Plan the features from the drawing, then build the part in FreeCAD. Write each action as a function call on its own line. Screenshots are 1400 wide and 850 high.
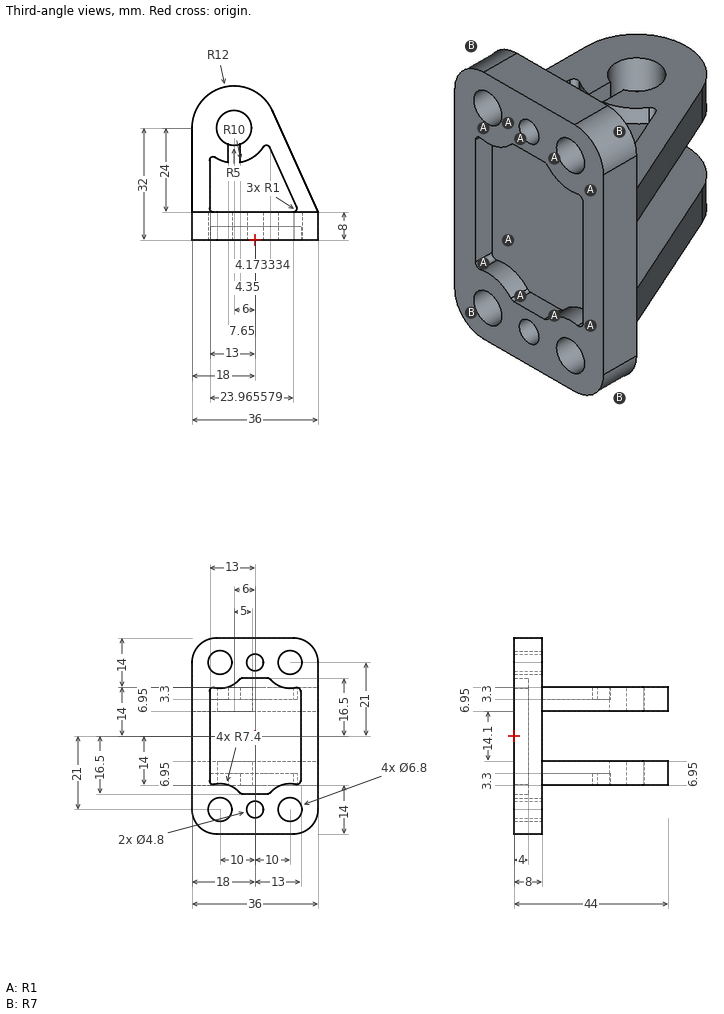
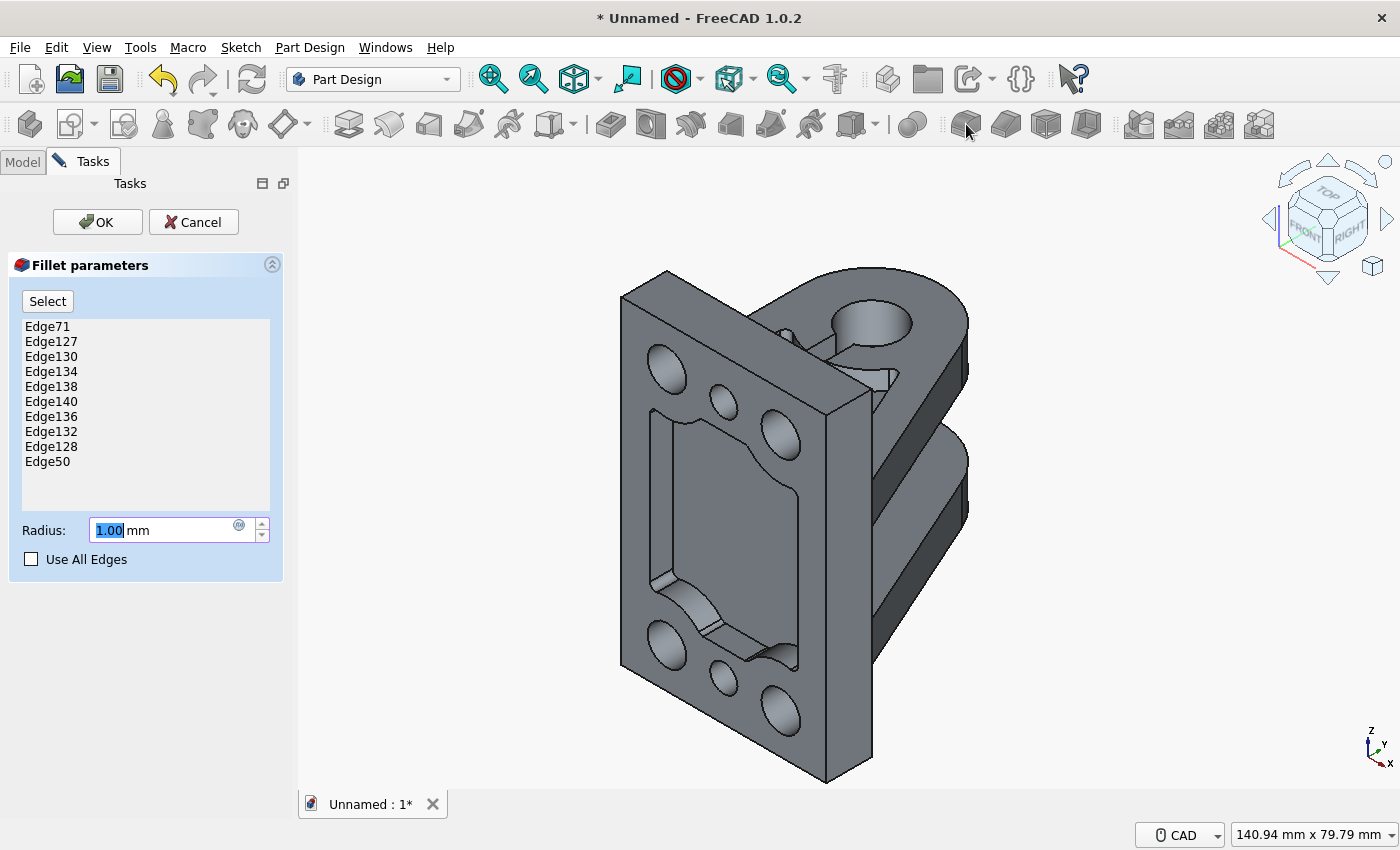
text(1)
key(Tab)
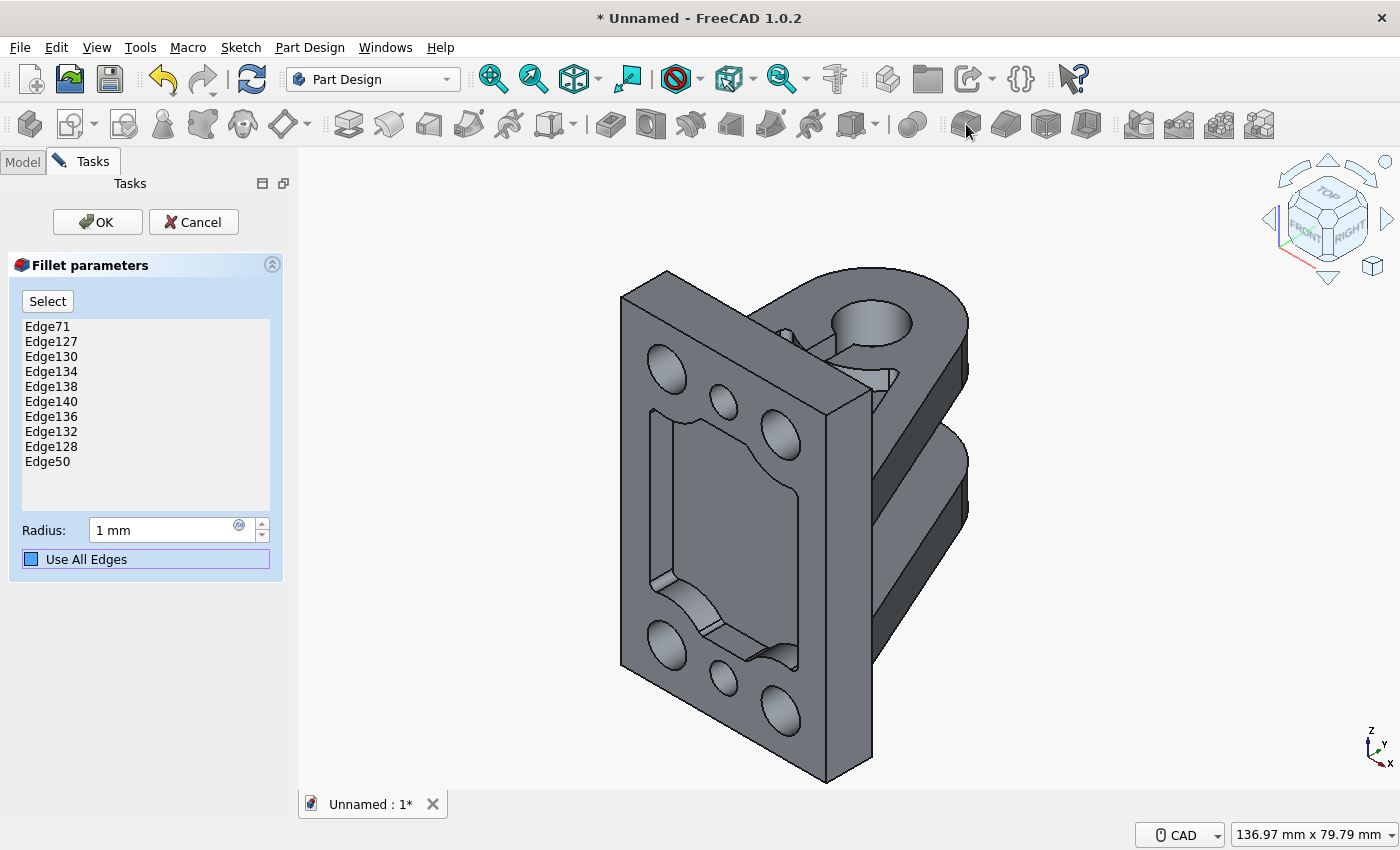
click(98, 222)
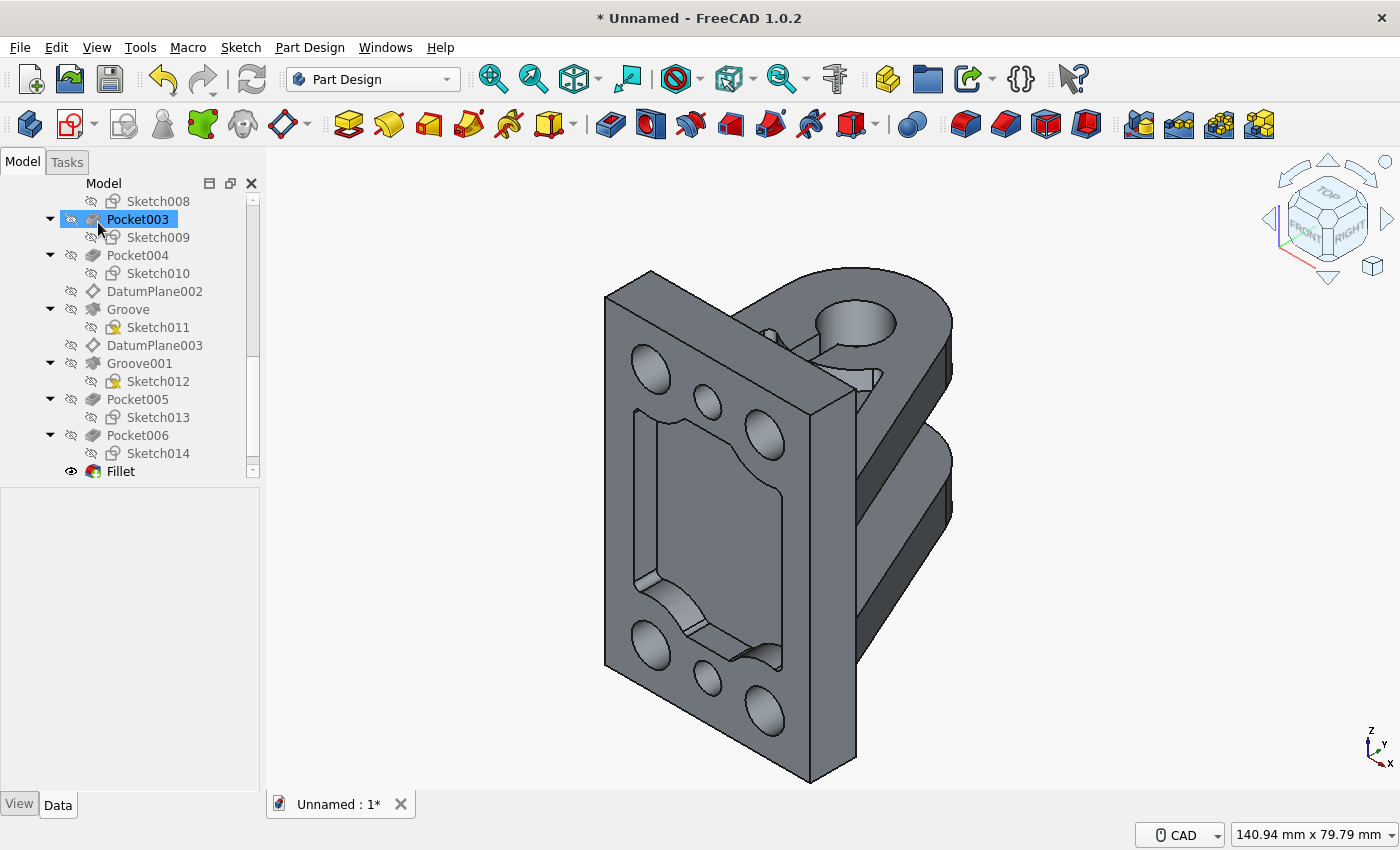
click(833, 401)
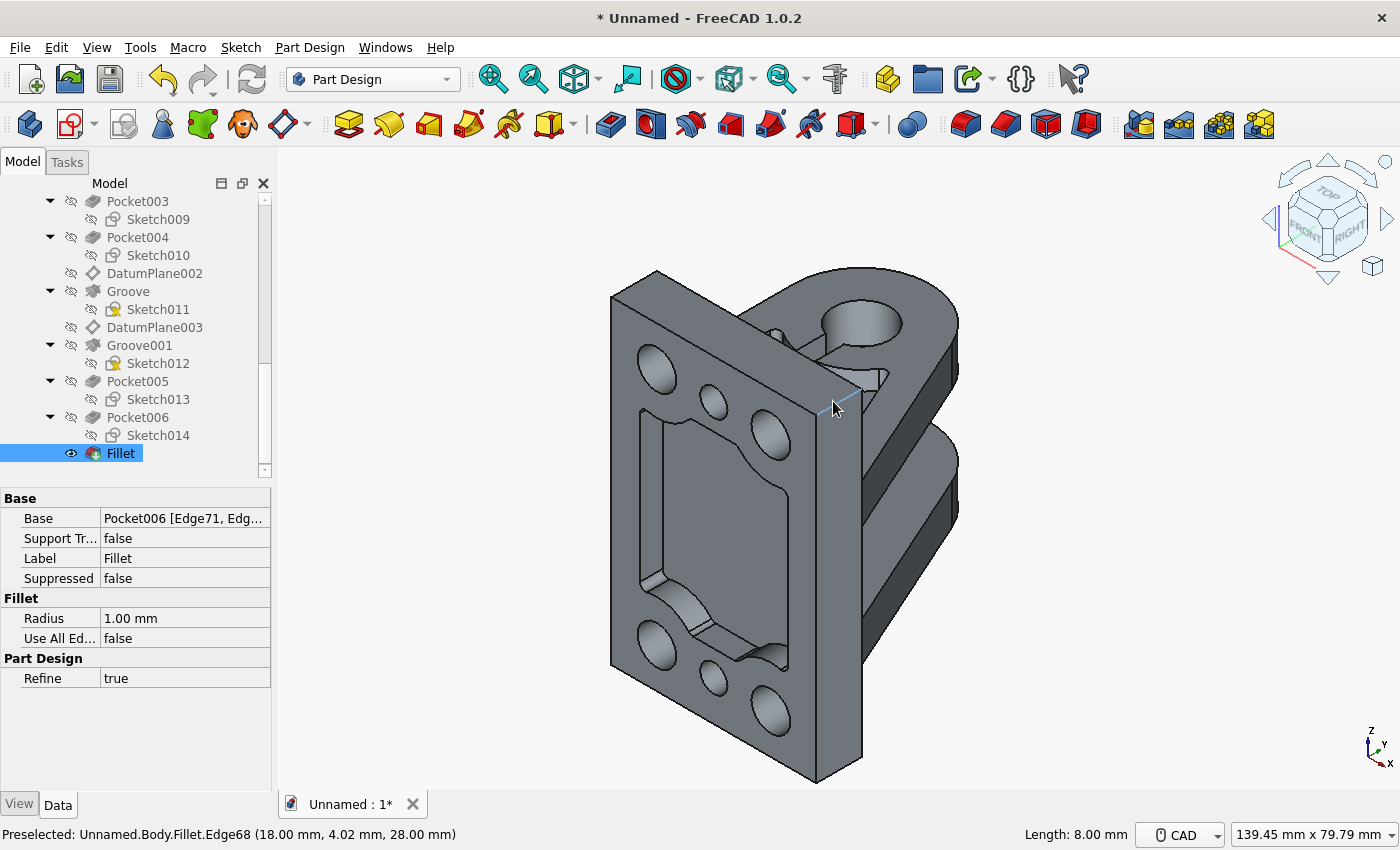
key(2)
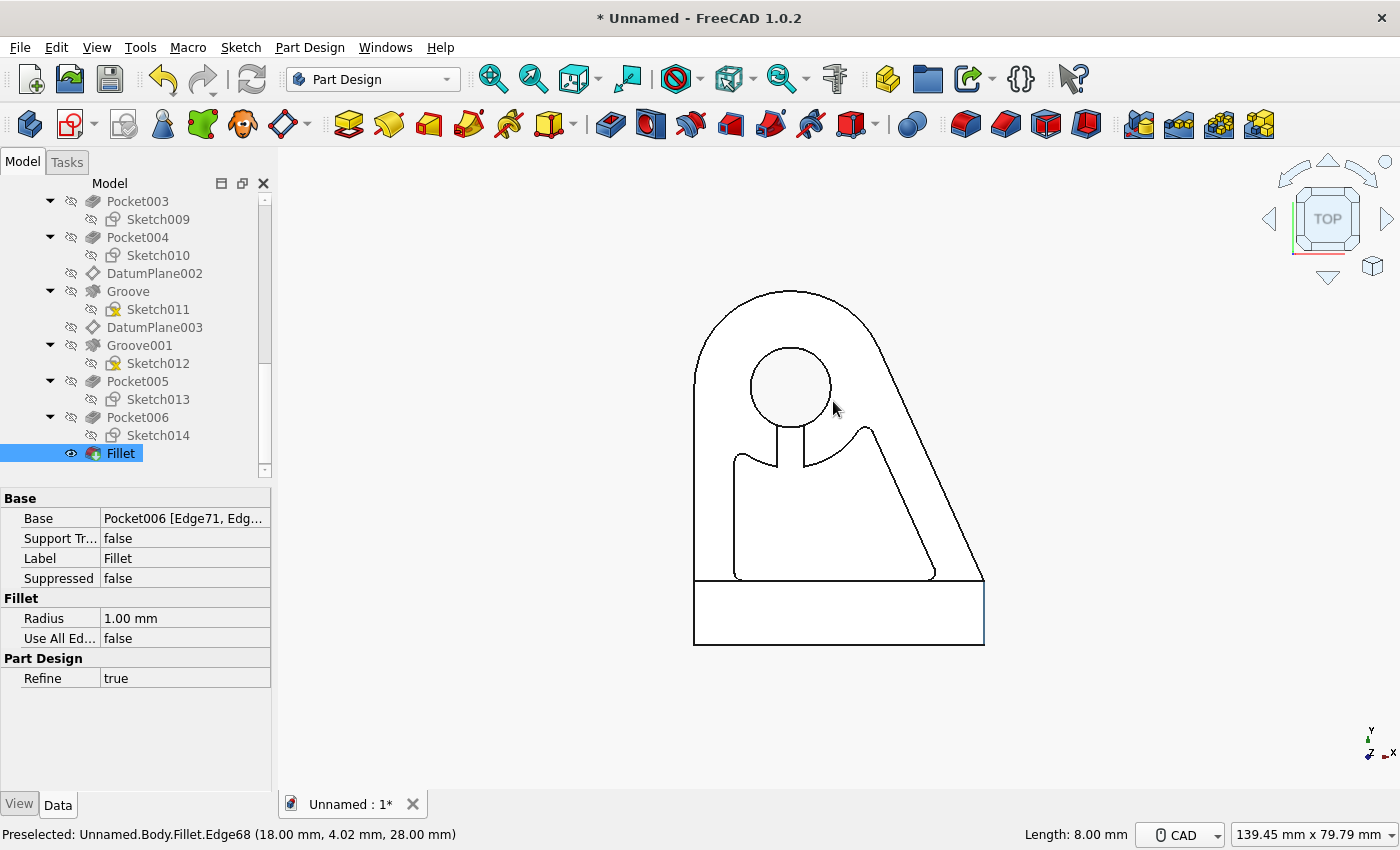
click(694, 612, ctrl)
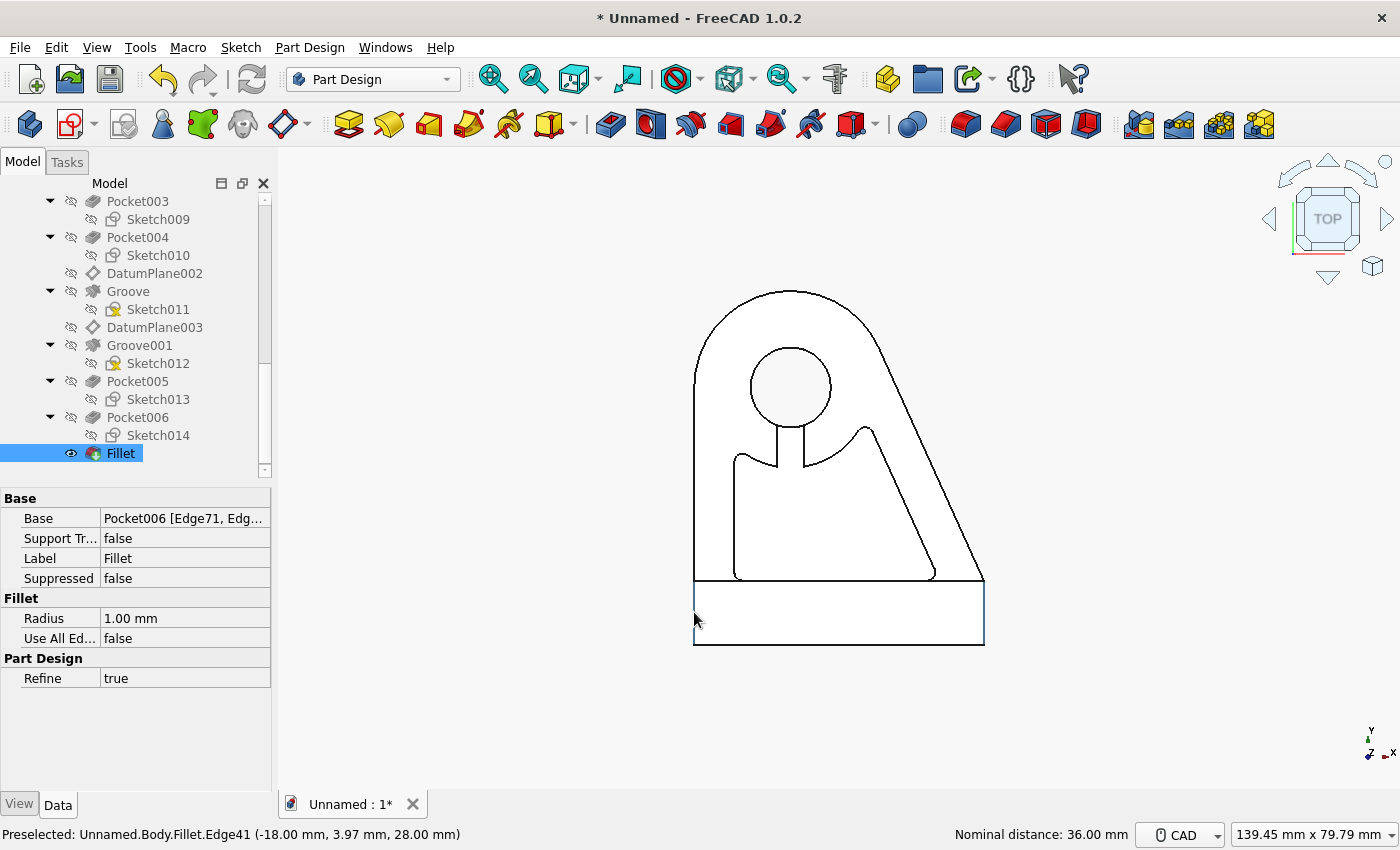
key(0)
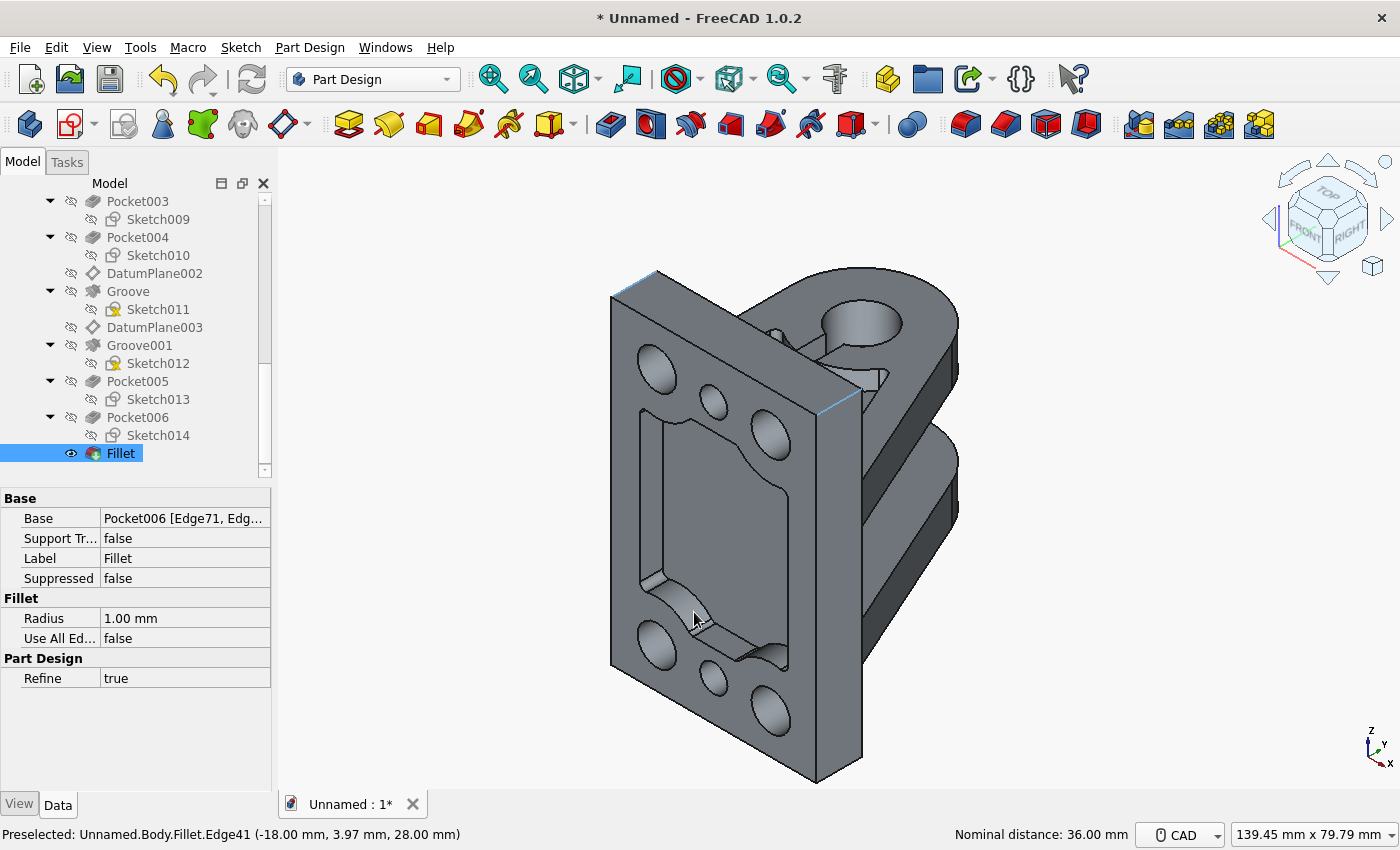
key(1)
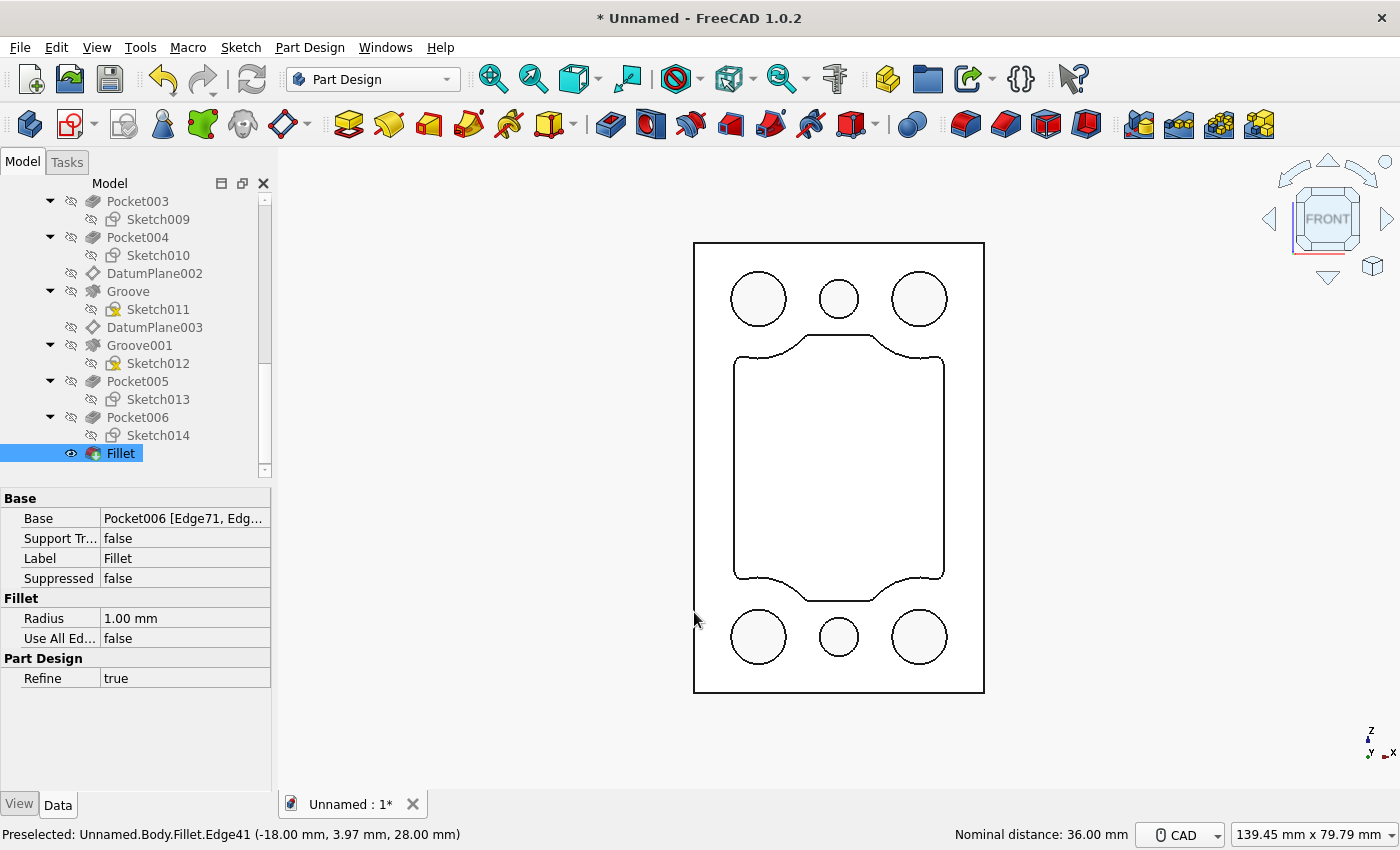
key(3)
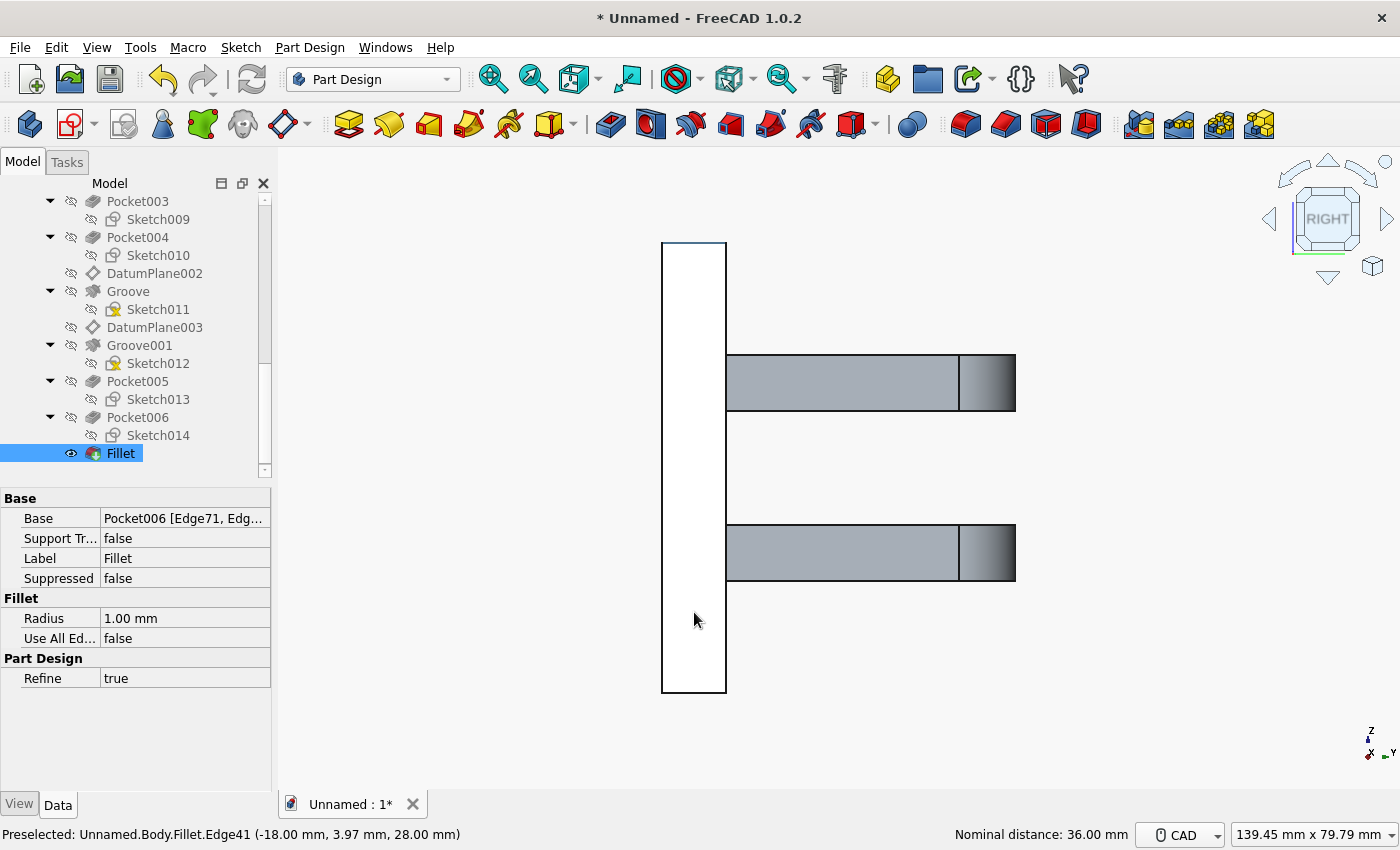
click(694, 692, ctrl)